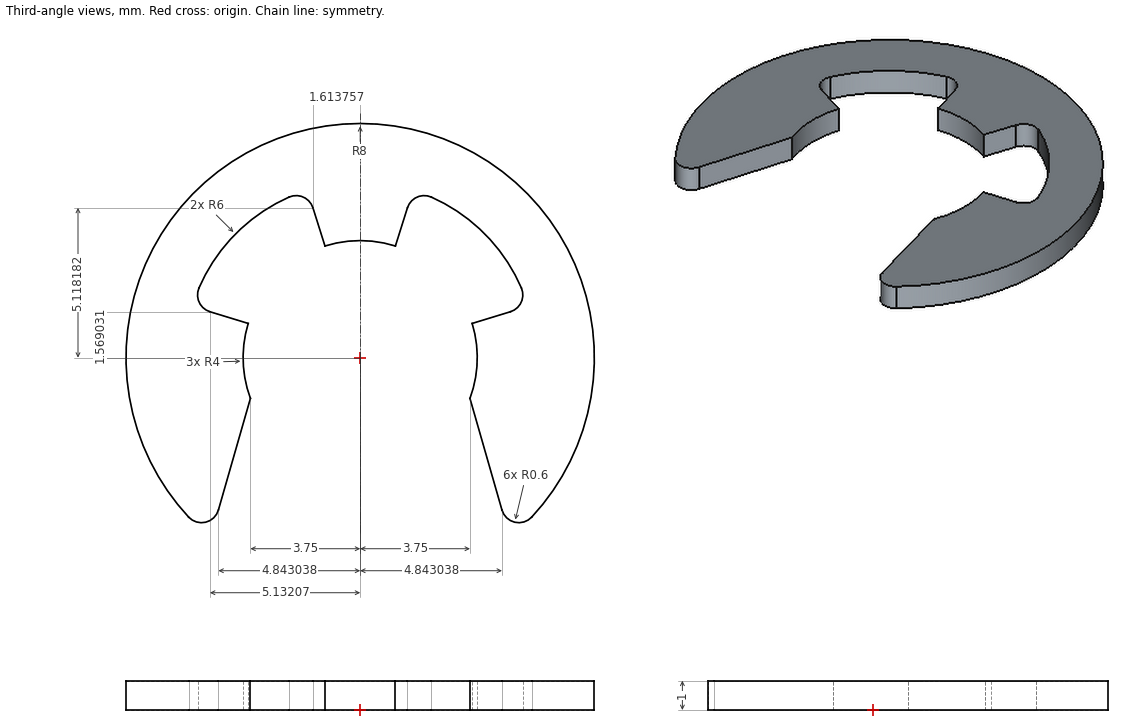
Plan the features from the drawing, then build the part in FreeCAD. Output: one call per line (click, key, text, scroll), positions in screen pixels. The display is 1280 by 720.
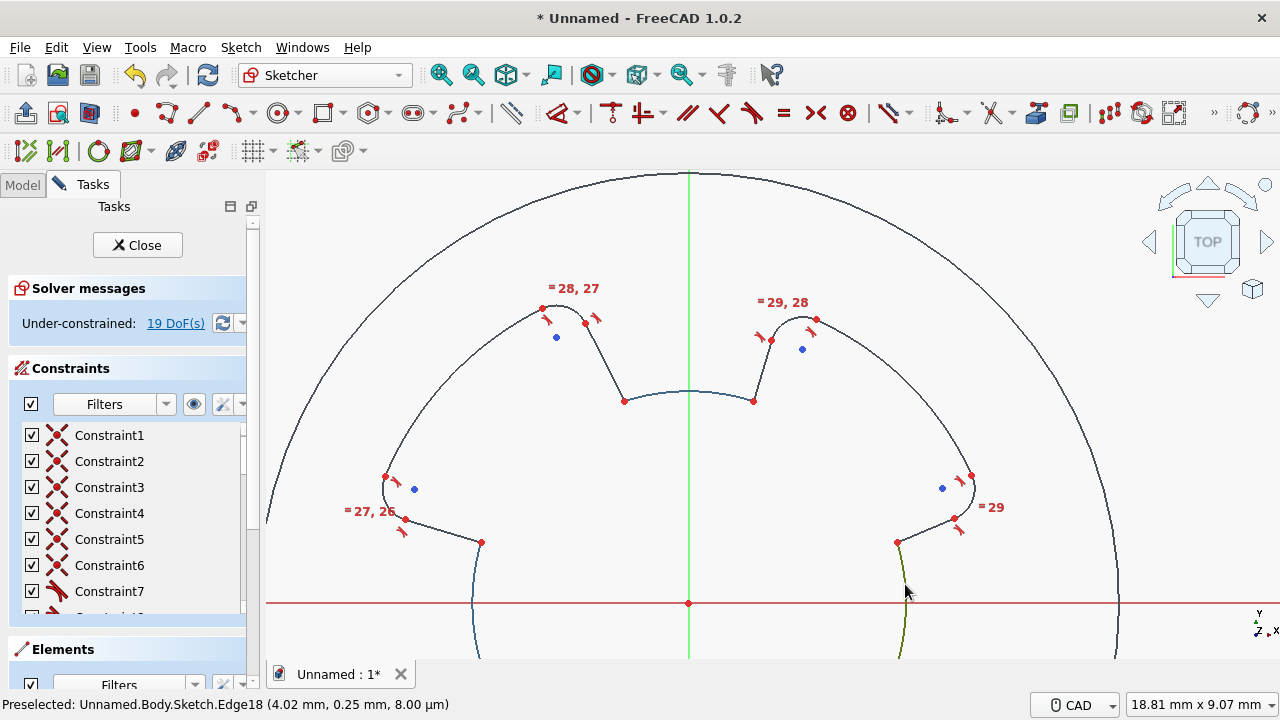
click(784, 114)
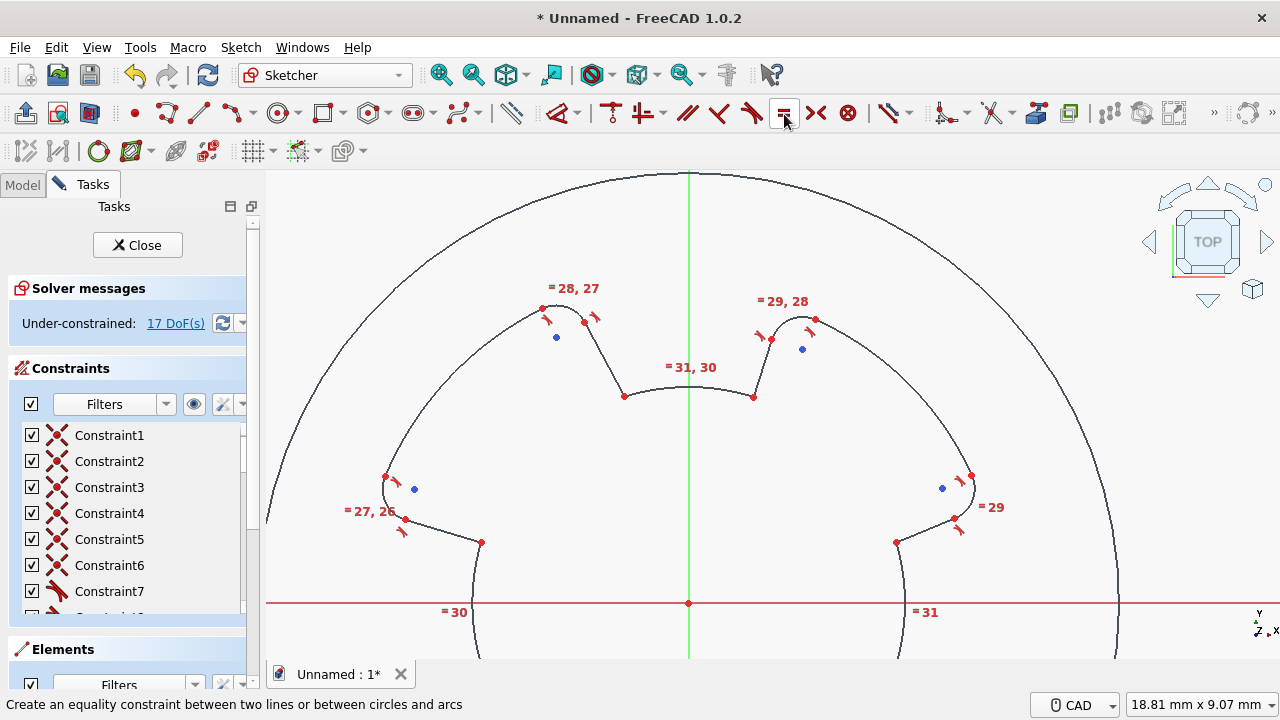
click(483, 347)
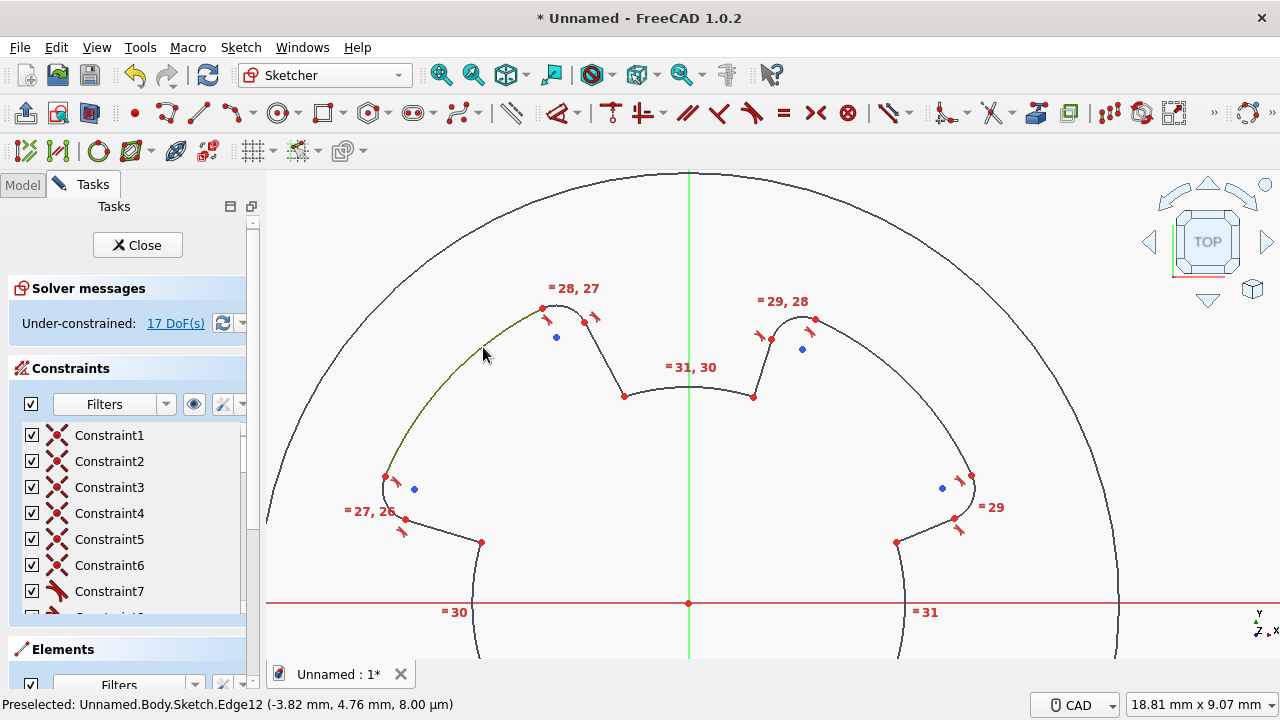
click(938, 417)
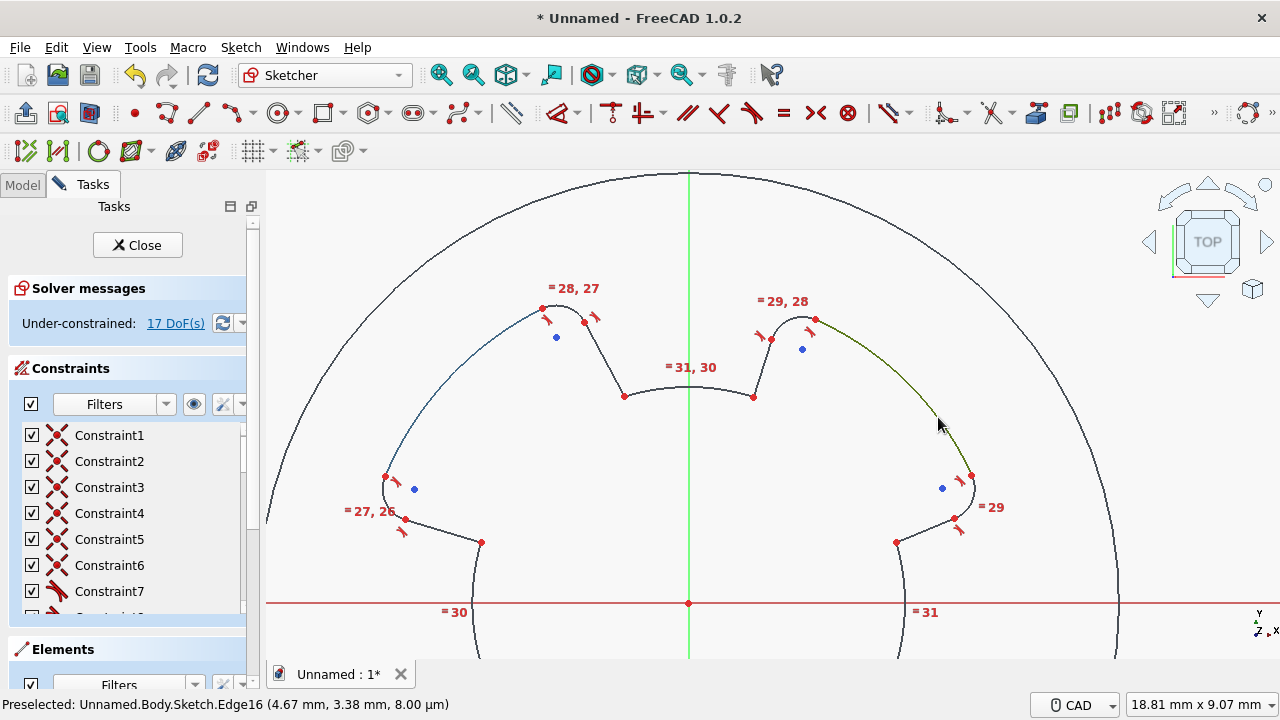
key(e)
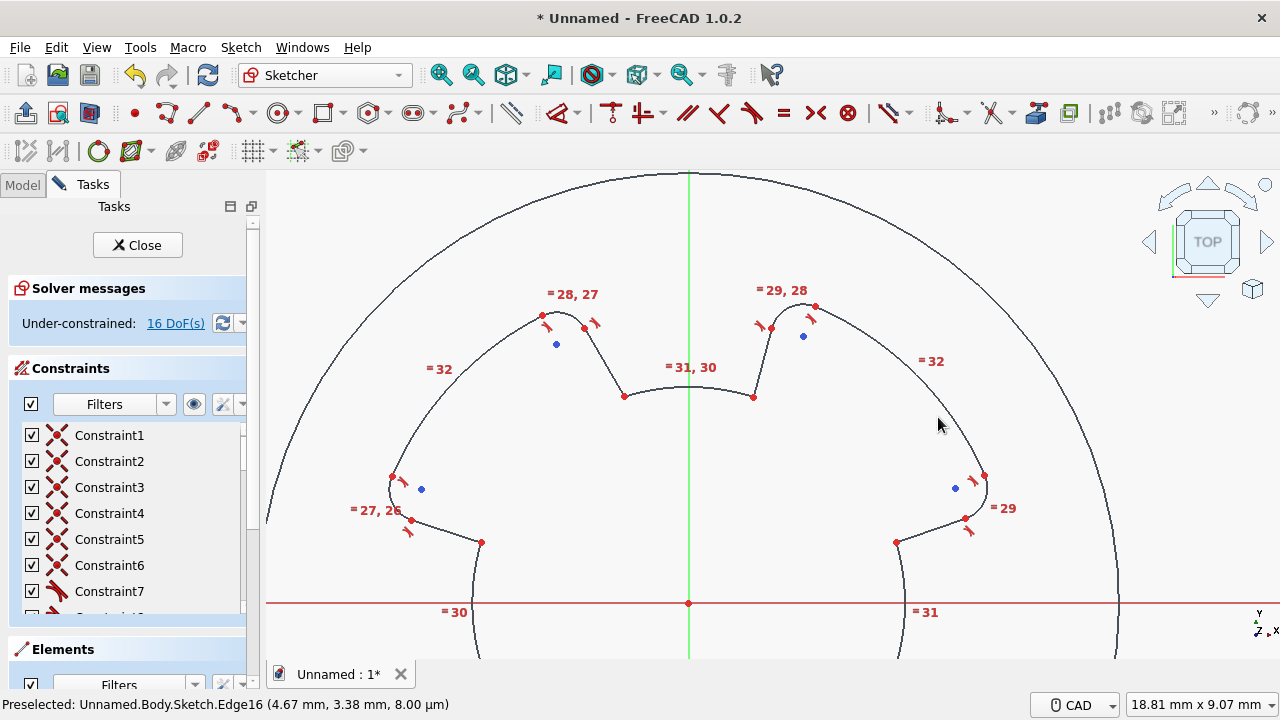
click(585, 328)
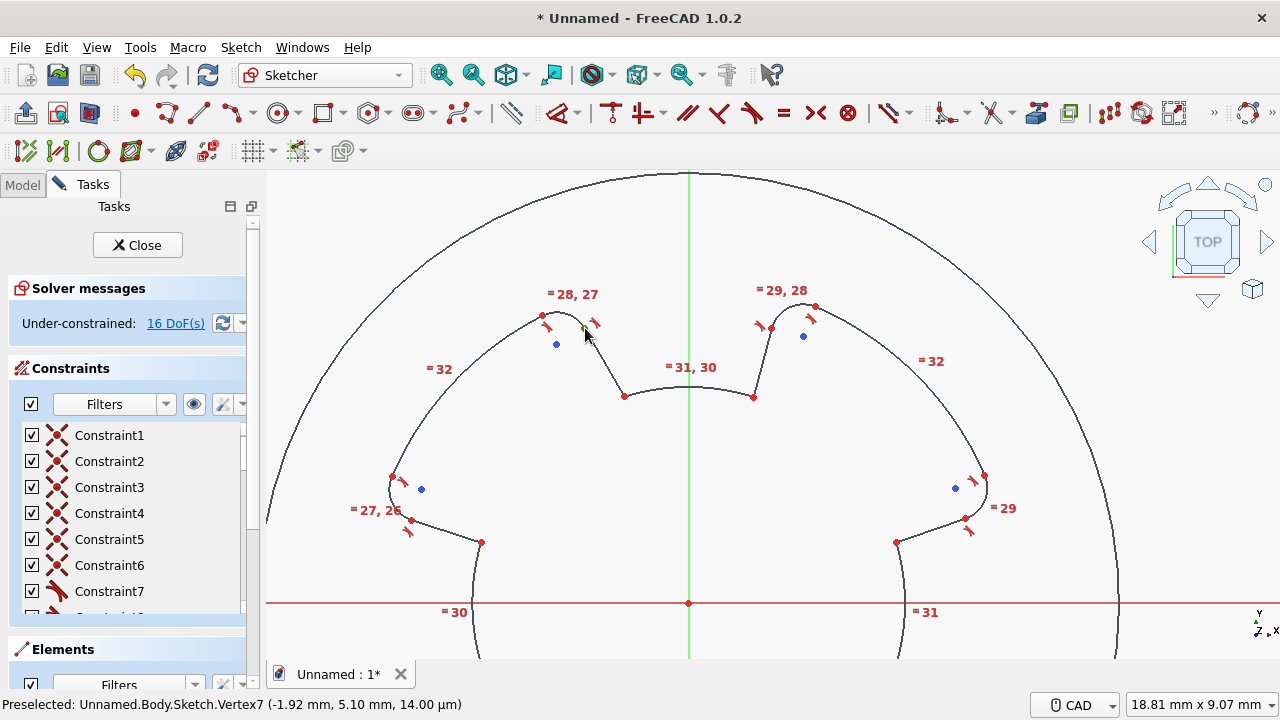
click(772, 328)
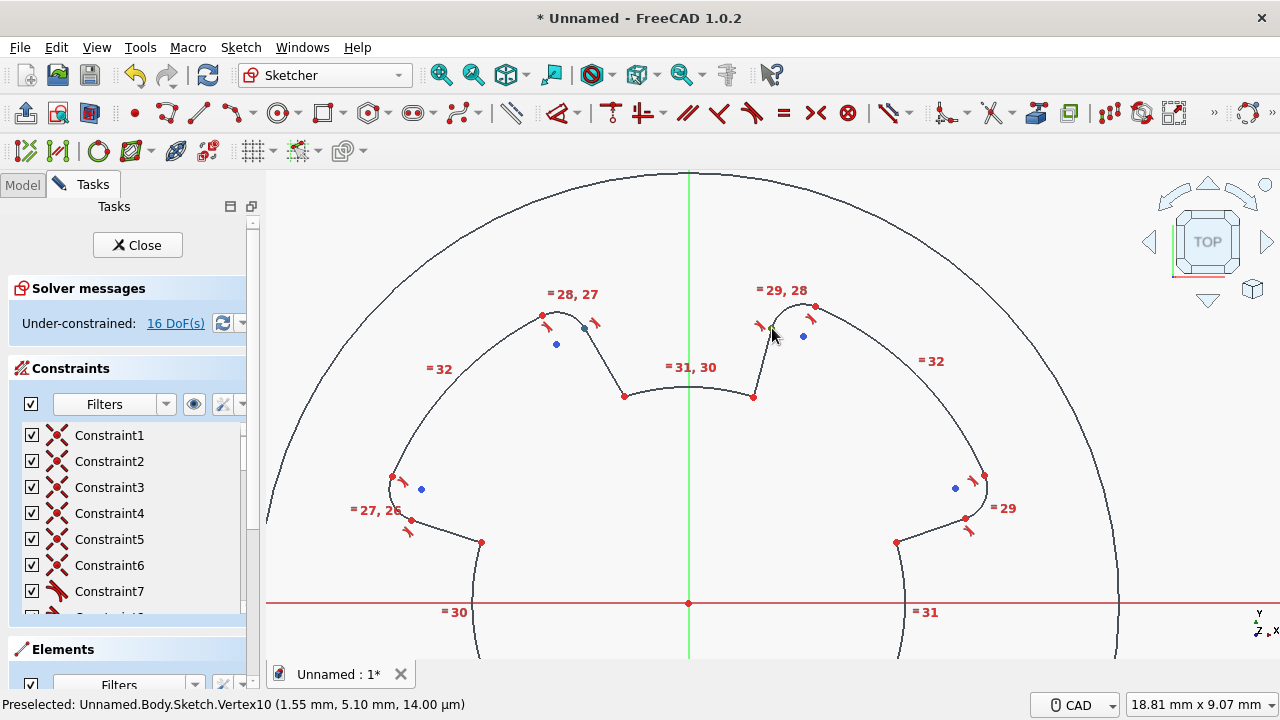
click(689, 569)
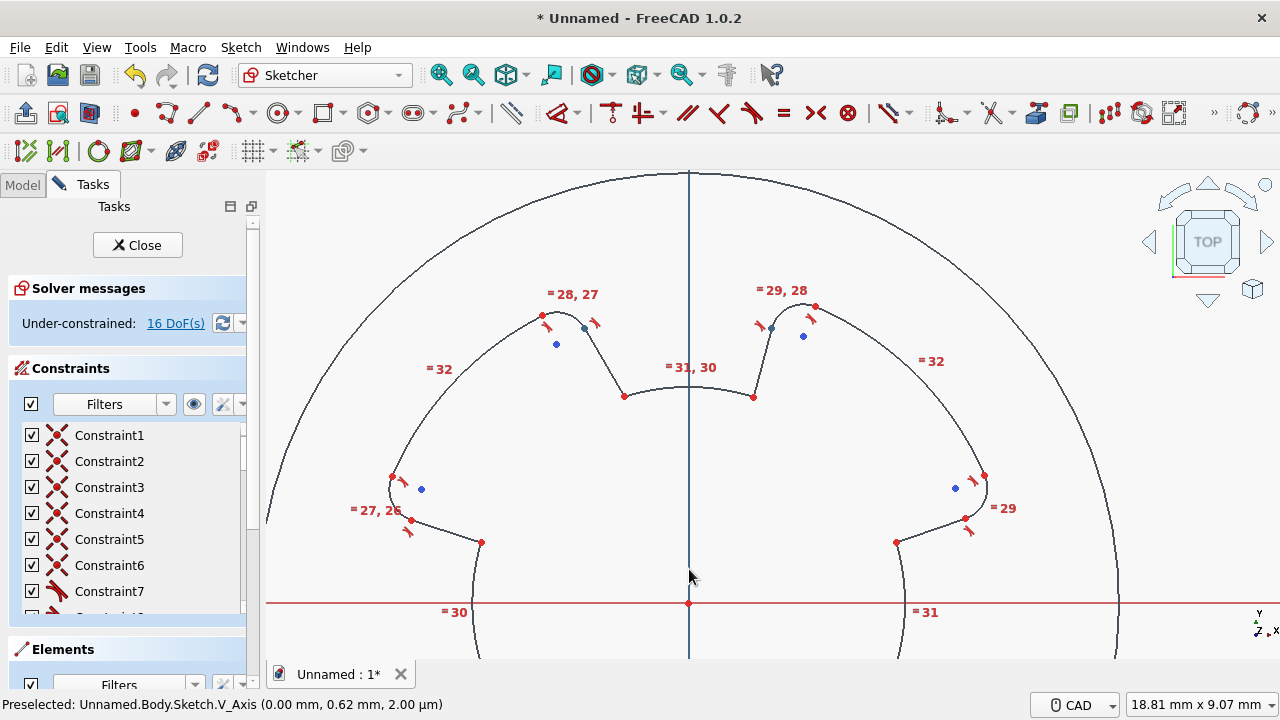
key(s)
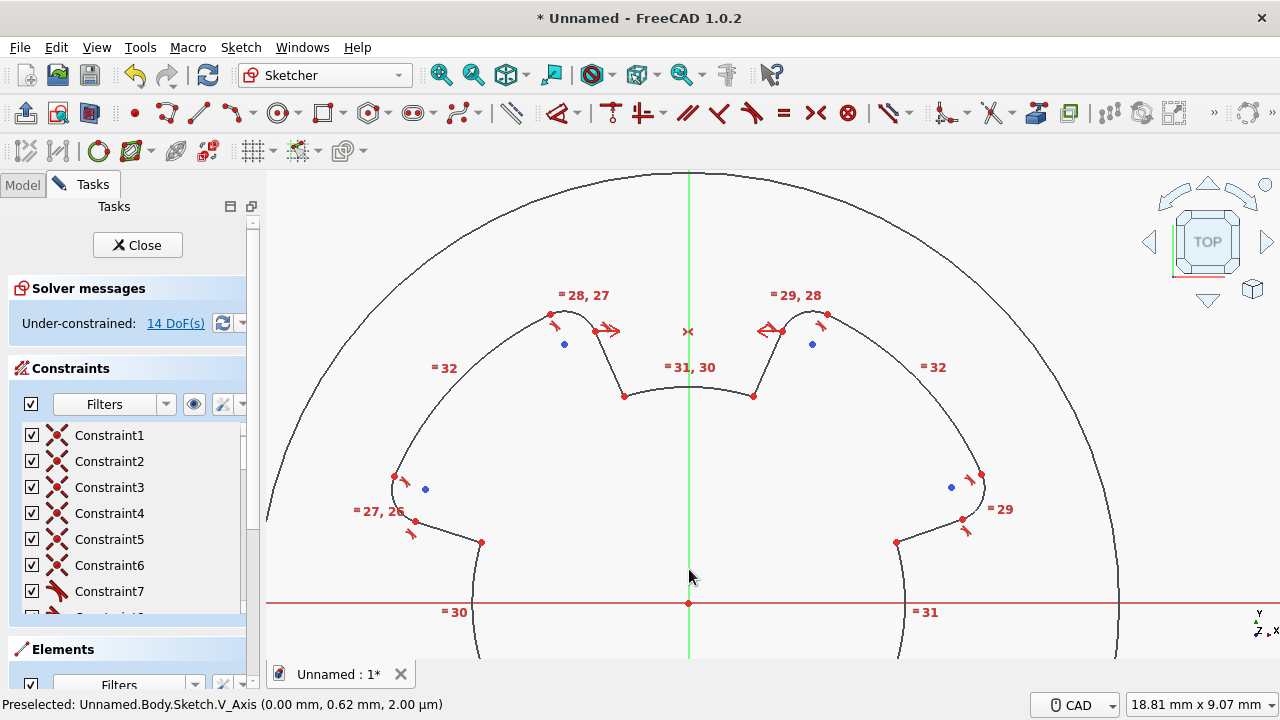
click(415, 522)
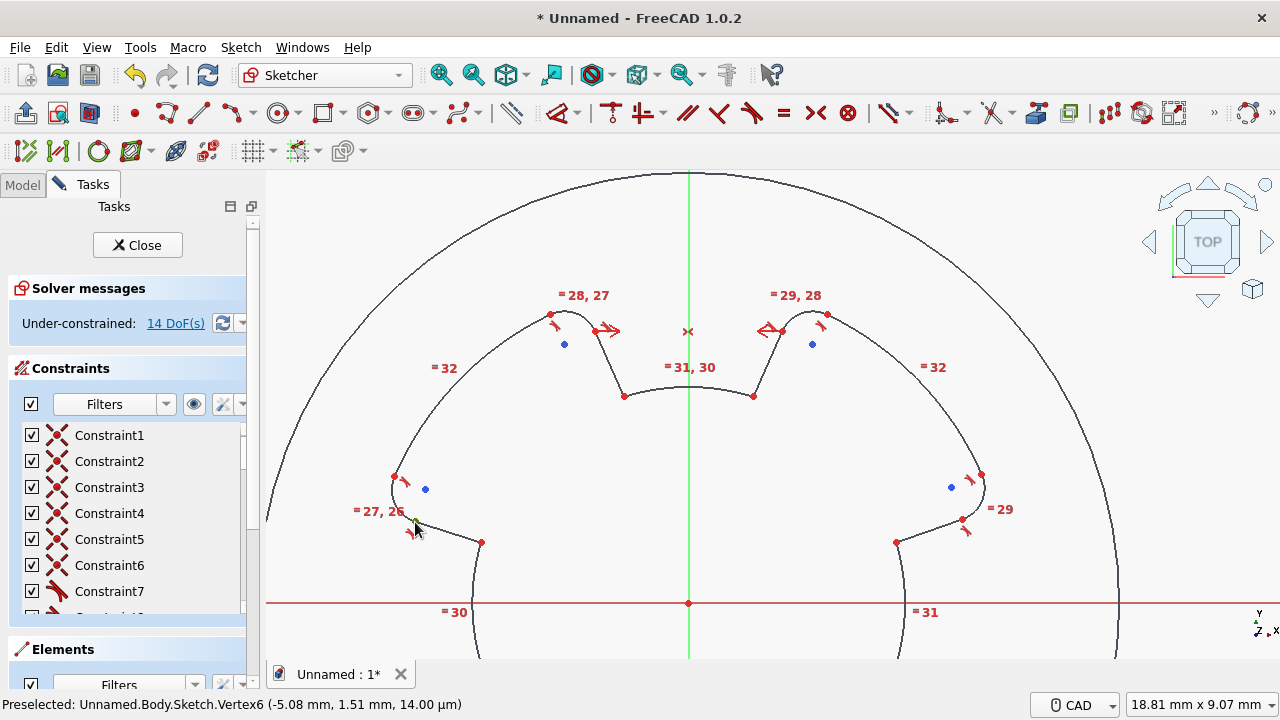
click(962, 519)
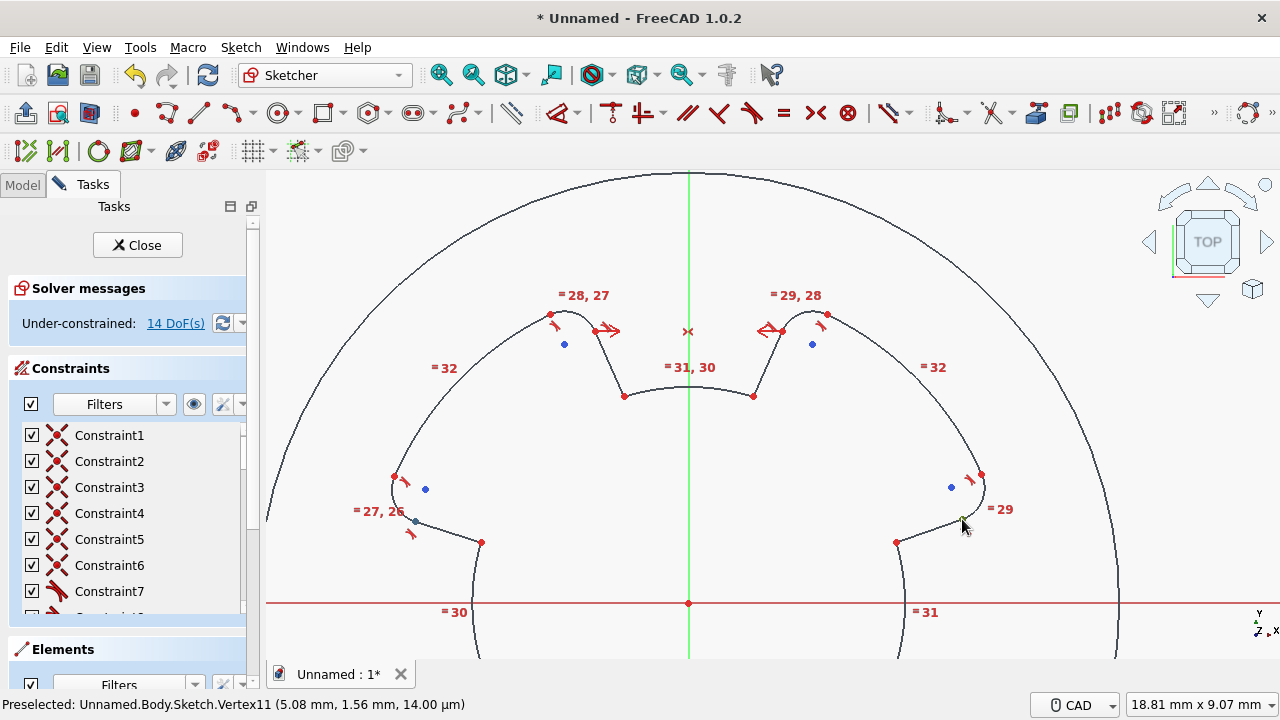
click(689, 569)